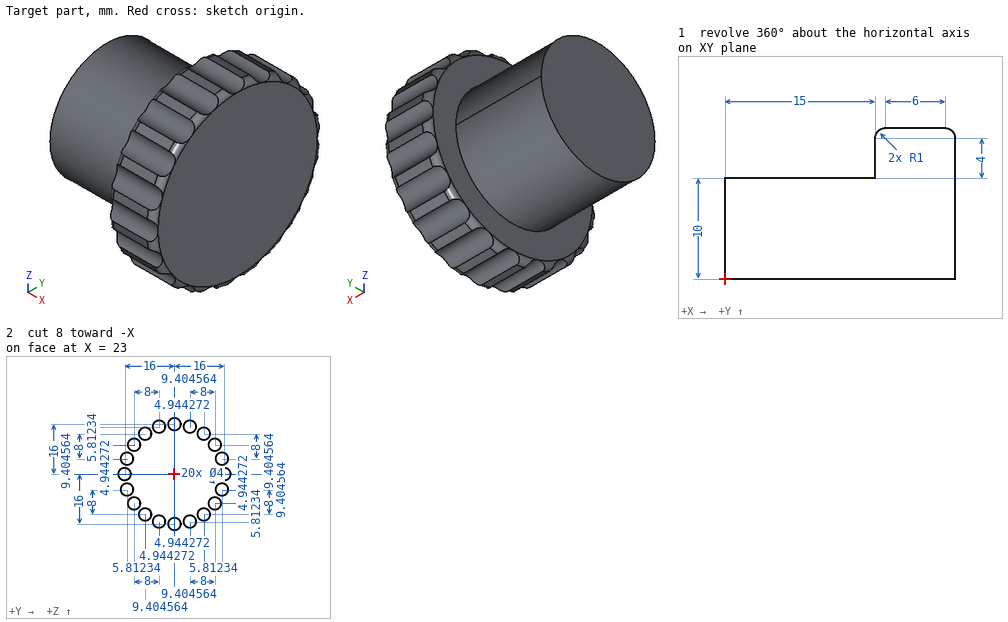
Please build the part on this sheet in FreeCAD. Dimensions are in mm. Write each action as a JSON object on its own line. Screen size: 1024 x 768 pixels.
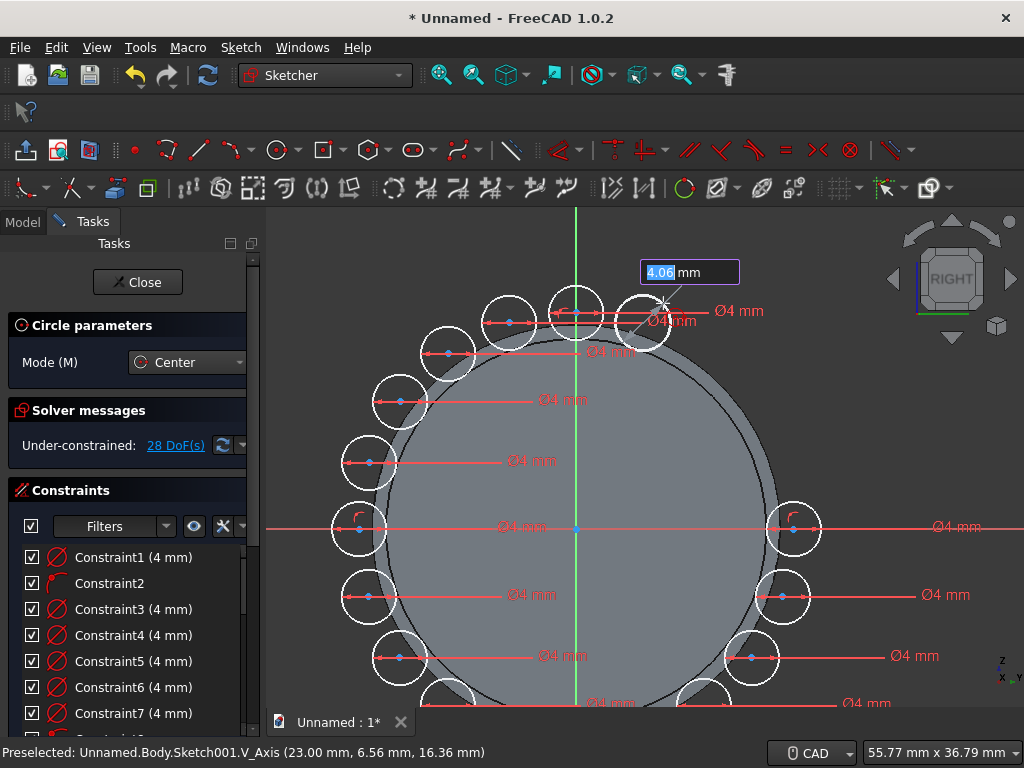
{"action": "type", "text": "4"}
{"action": "key", "text": "Return"}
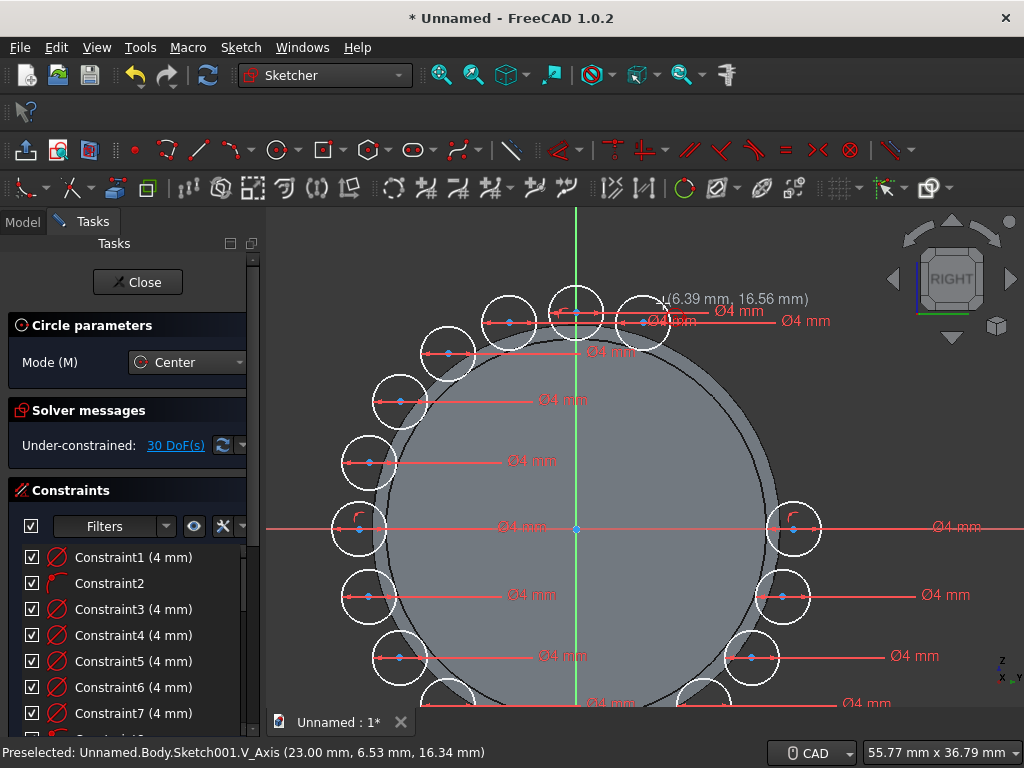
{"action": "left_click", "coordinate": [704, 353]}
{"action": "mouse_move", "coordinate": [723, 334]}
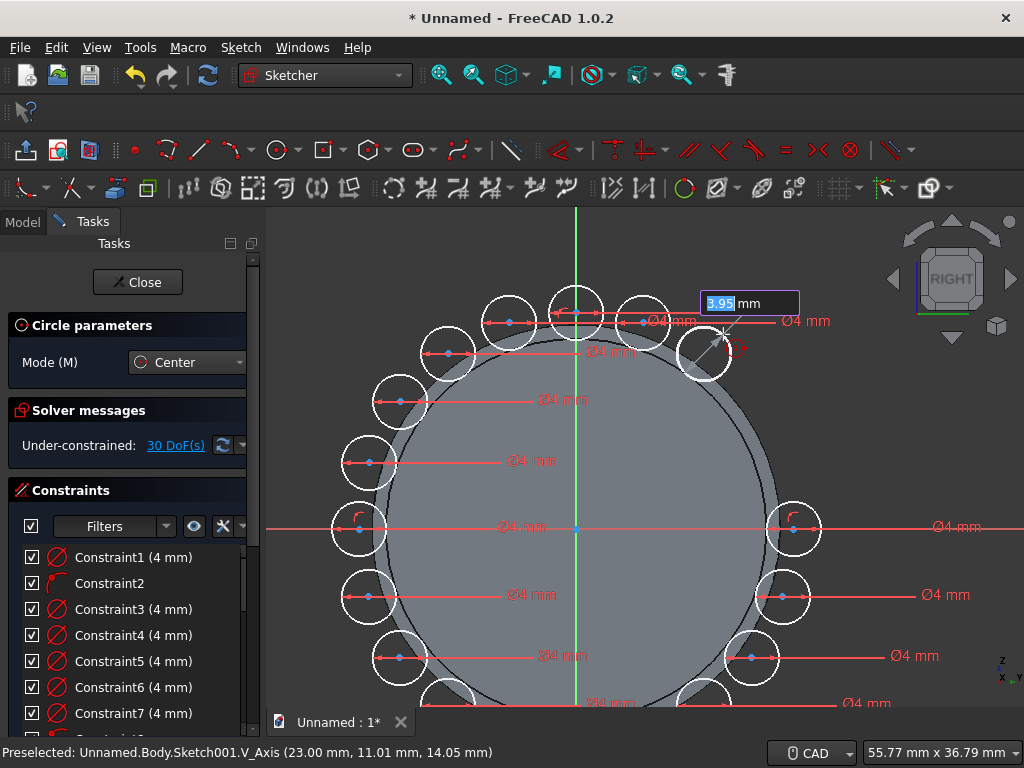
{"action": "type", "text": "4"}
{"action": "key", "text": "Return"}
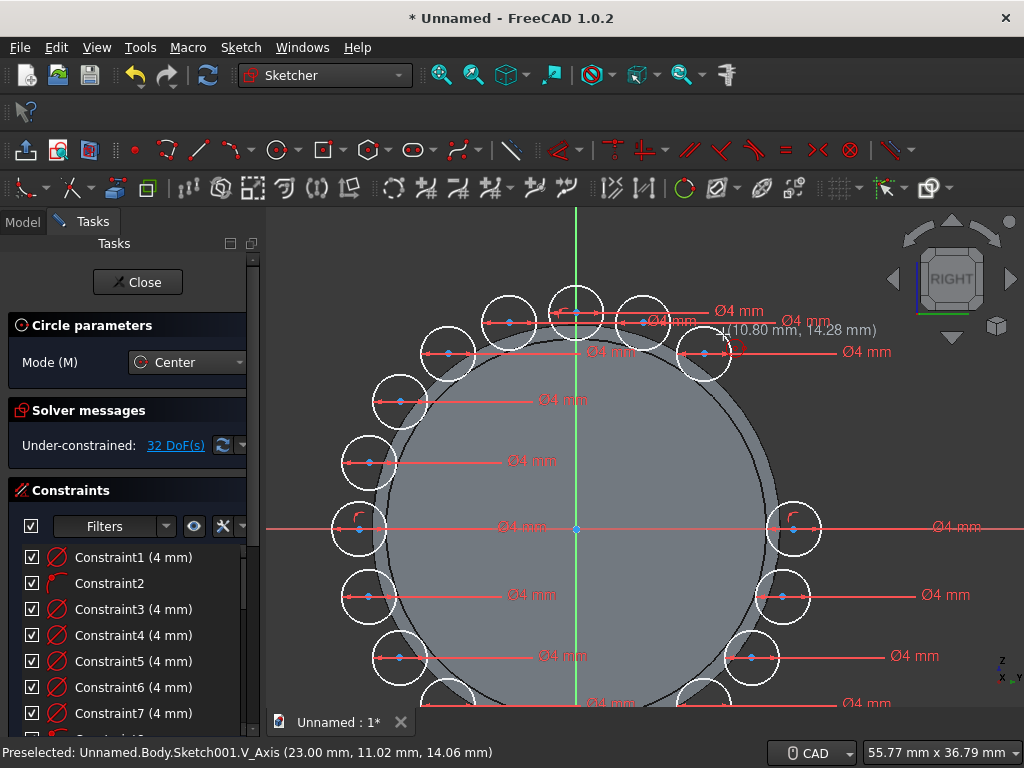
{"action": "left_click", "coordinate": [752, 401]}
{"action": "mouse_move", "coordinate": [771, 382]}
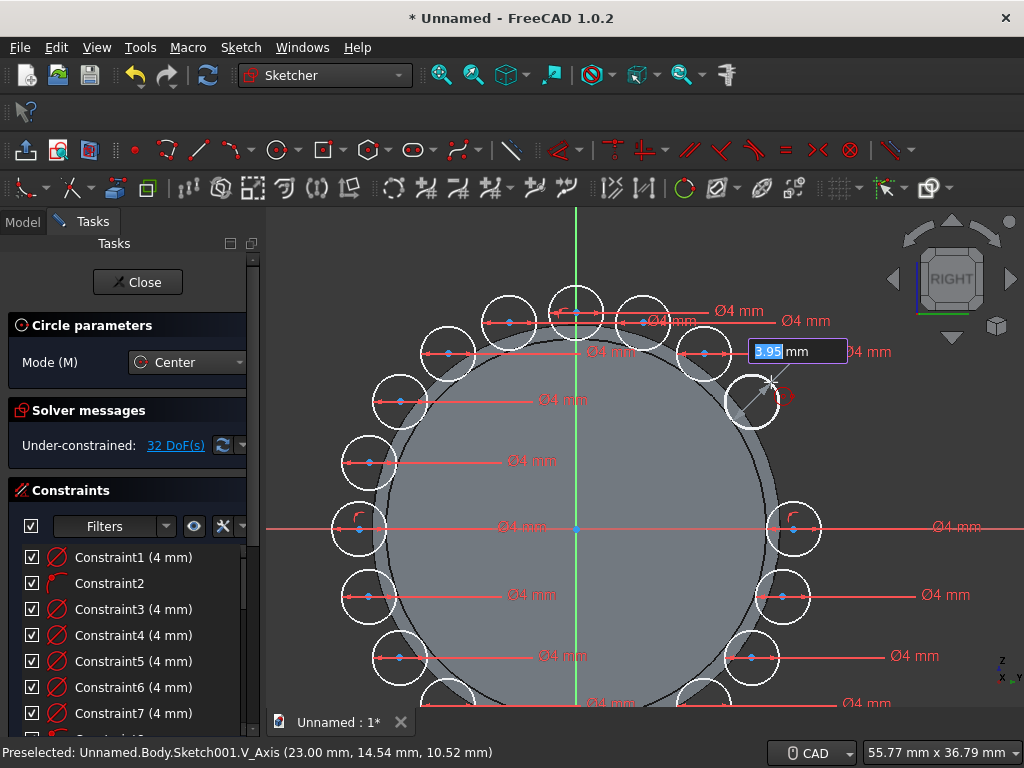
{"action": "type", "text": "4"}
{"action": "key", "text": "Return"}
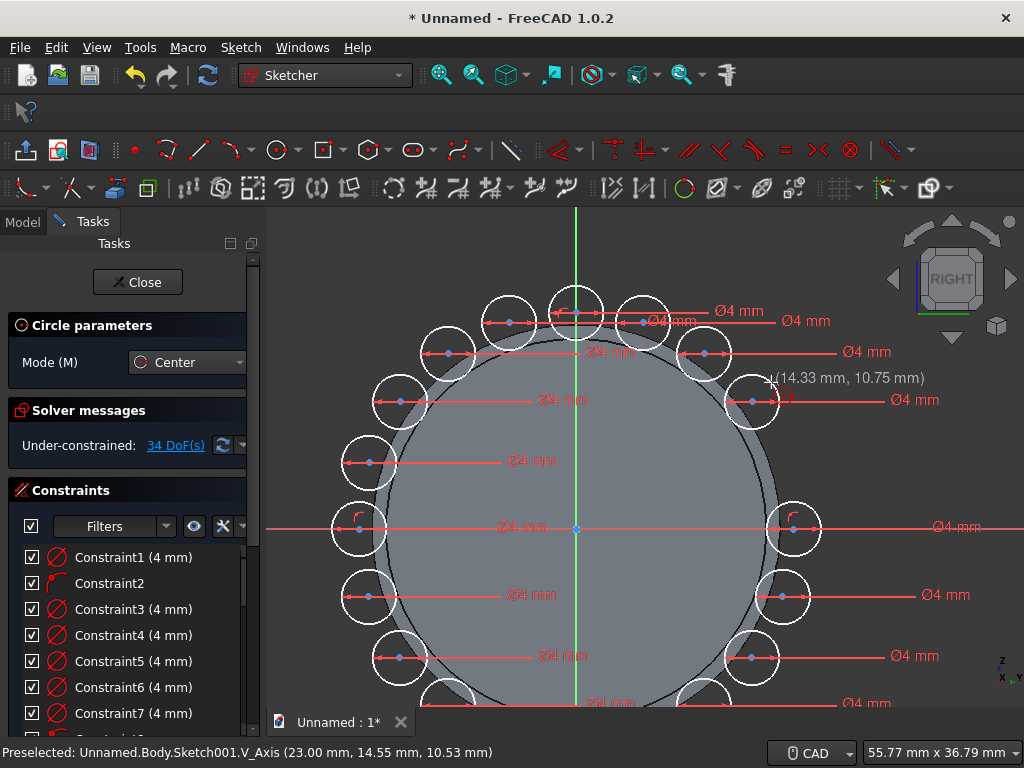
{"action": "left_click", "coordinate": [783, 462]}
{"action": "mouse_move", "coordinate": [802, 443]}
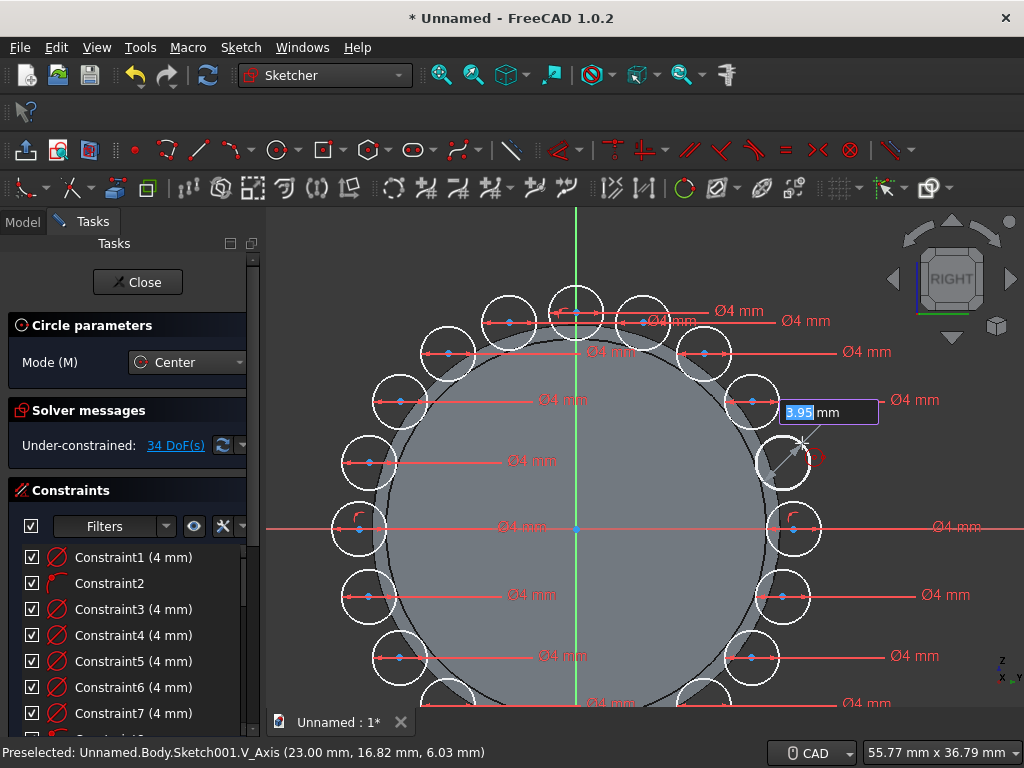
{"action": "type", "text": "4"}
{"action": "key", "text": "Return"}
{"action": "key", "text": "Escape"}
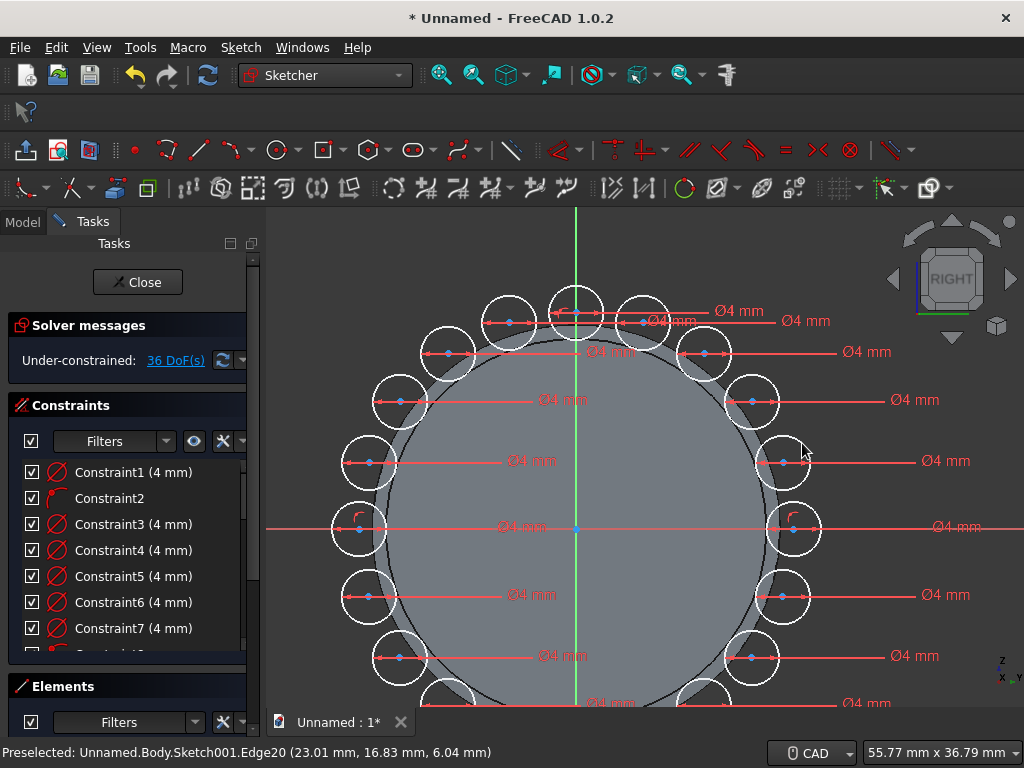
{"action": "scroll", "coordinate": [577, 310], "scroll_direction": "down", "scroll_amount": 2}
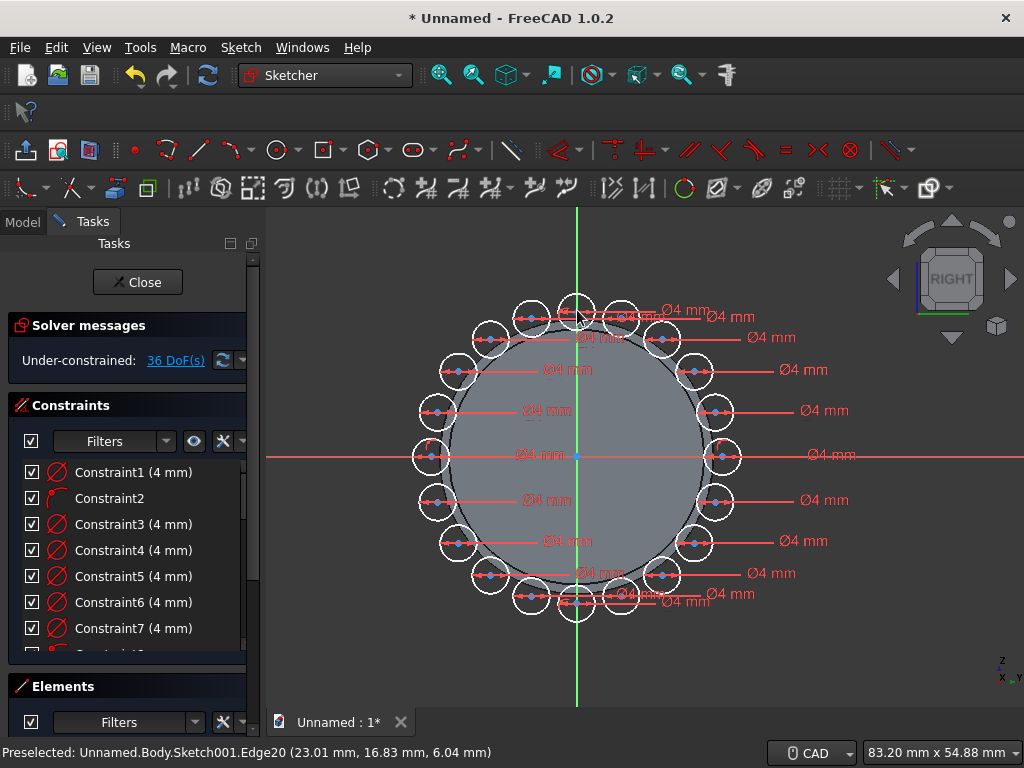
{"action": "left_click", "coordinate": [621, 596]}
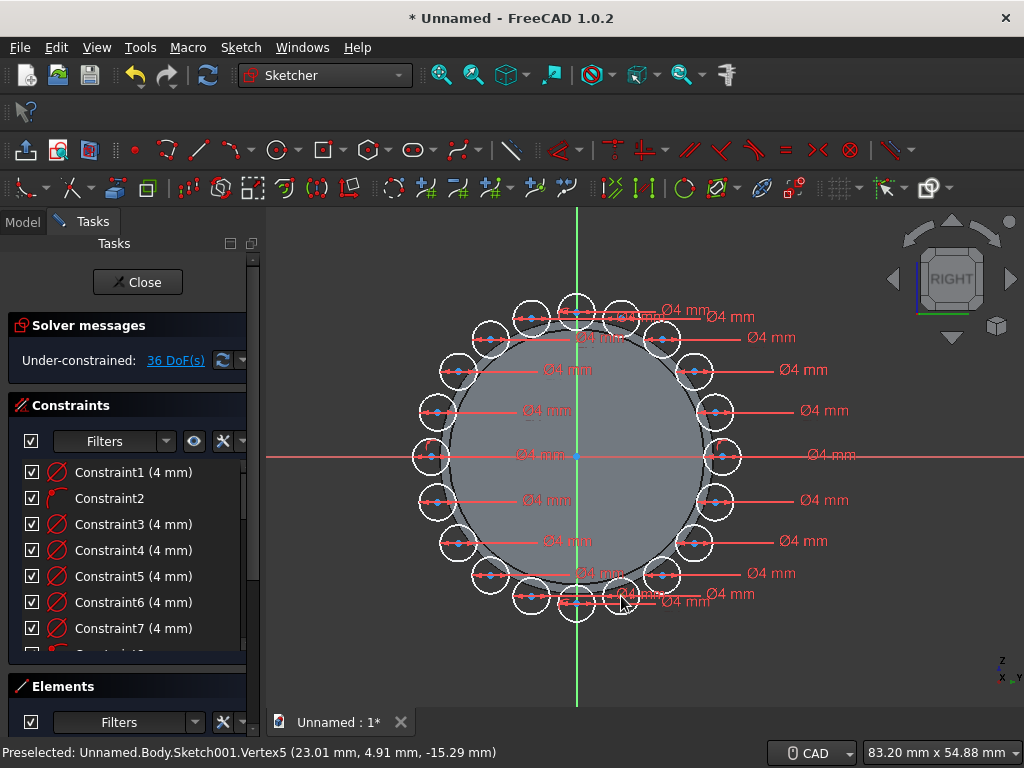
{"action": "left_click", "coordinate": [531, 596]}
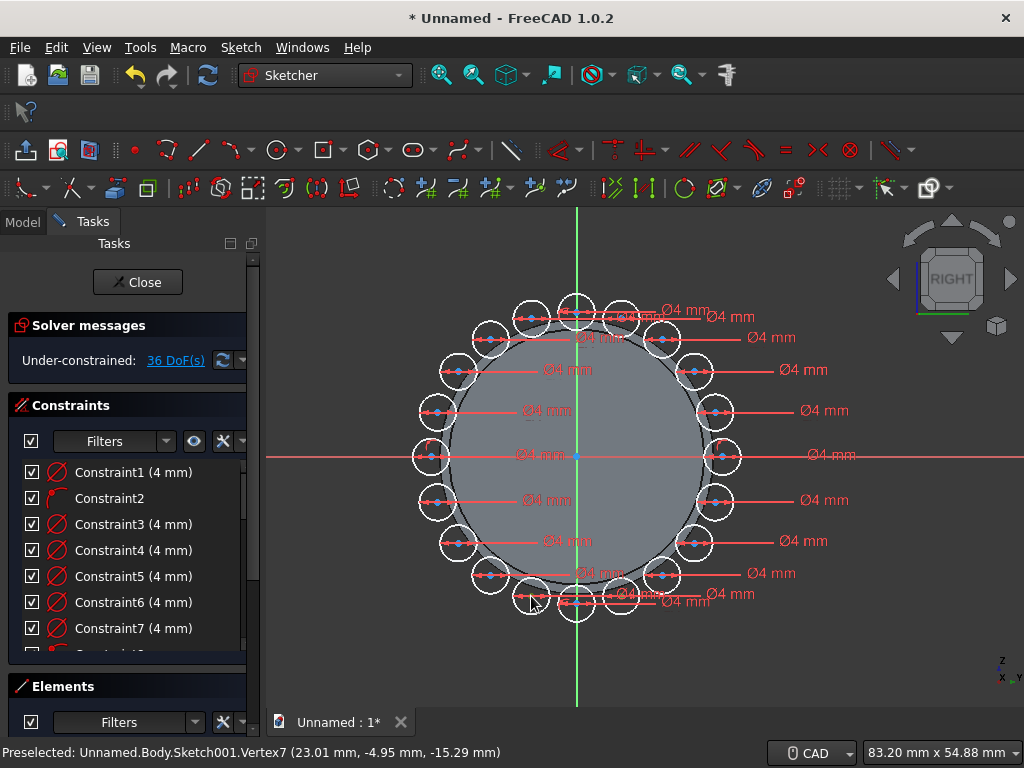
{"action": "key", "text": "h"}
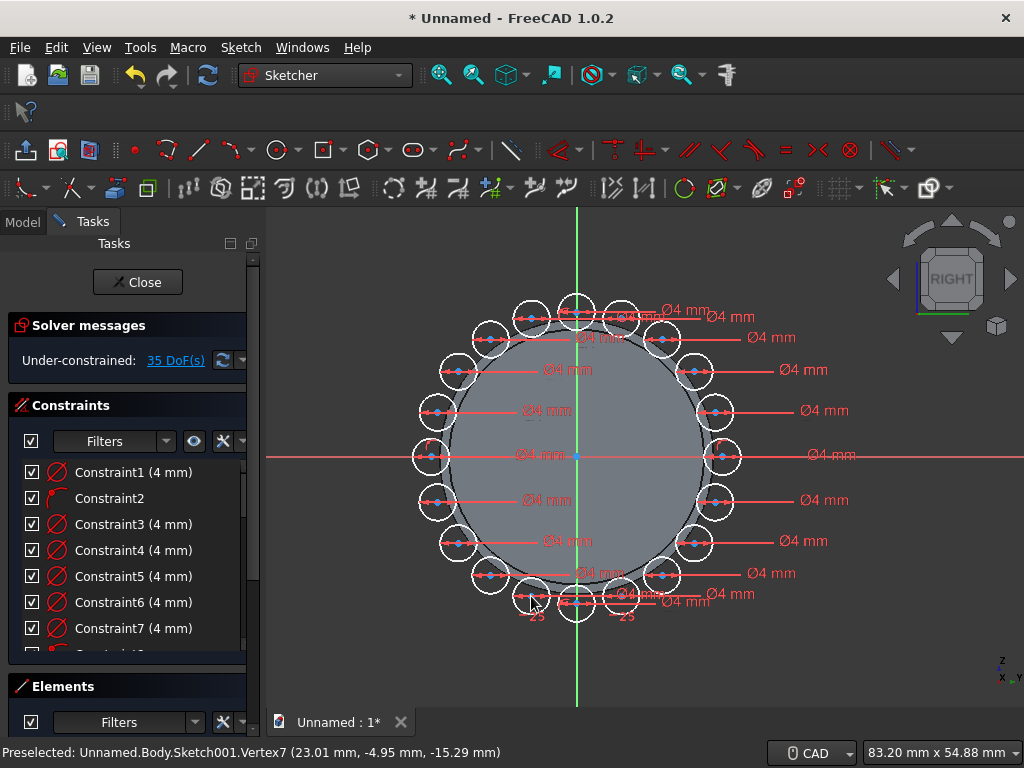
{"action": "left_click", "coordinate": [662, 575]}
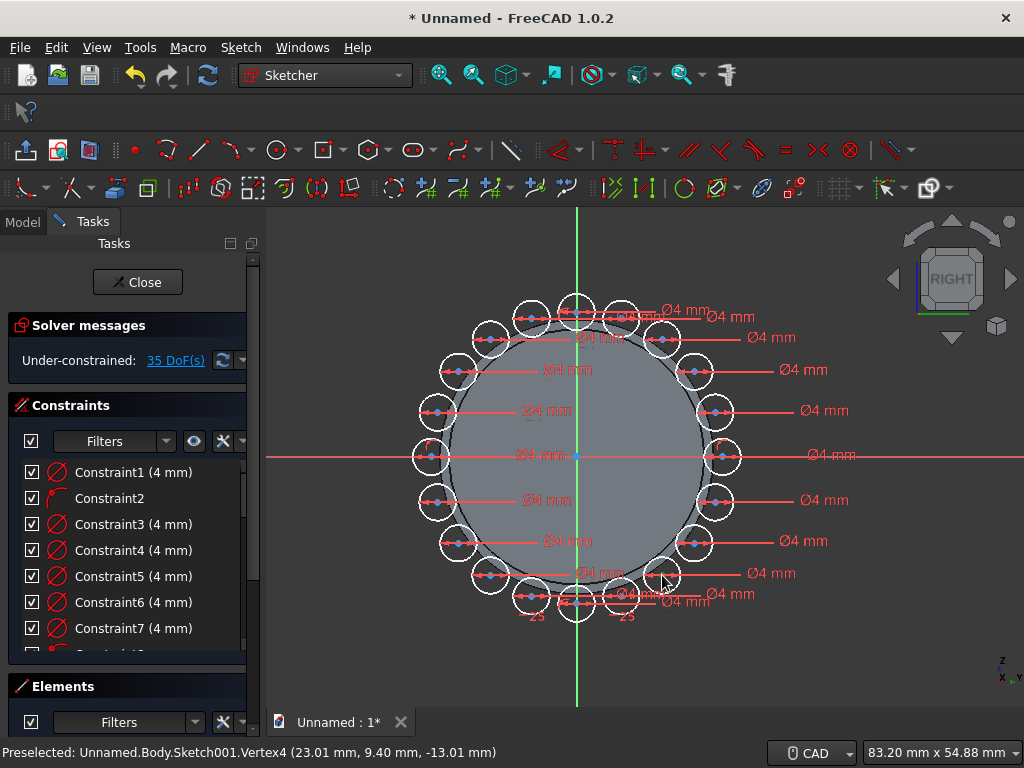
{"action": "left_click", "coordinate": [491, 575]}